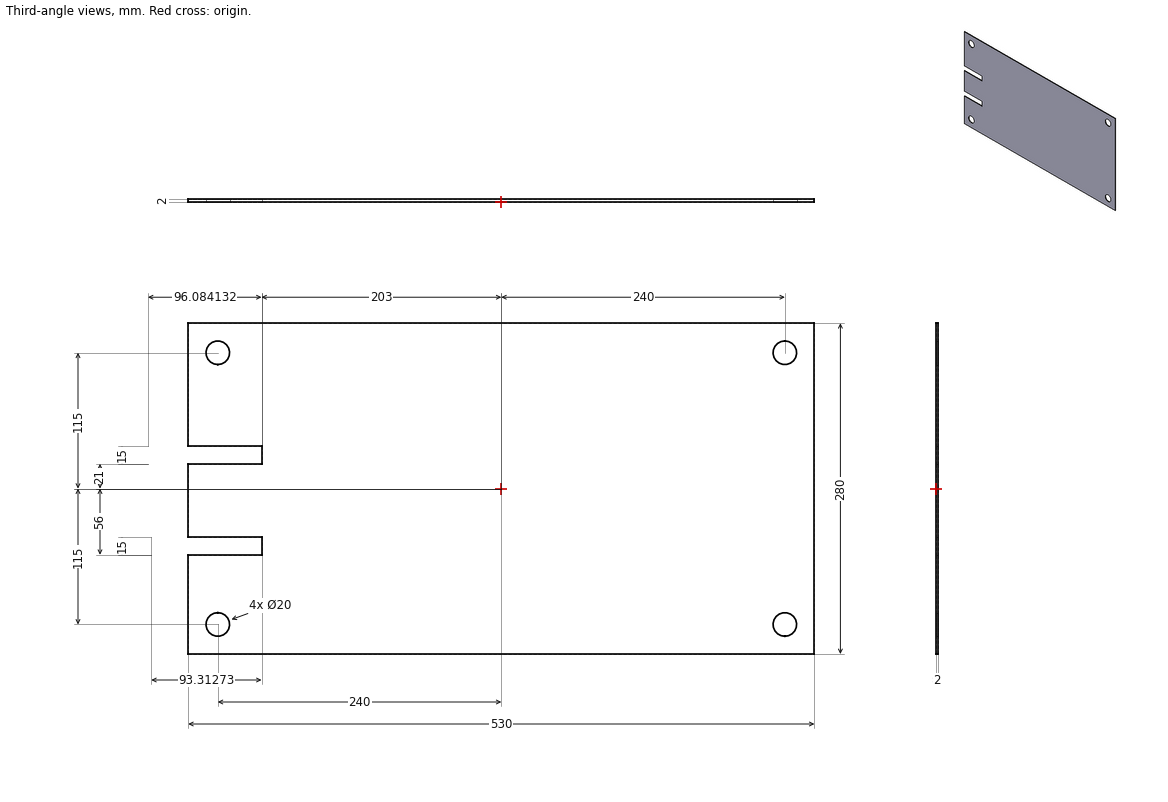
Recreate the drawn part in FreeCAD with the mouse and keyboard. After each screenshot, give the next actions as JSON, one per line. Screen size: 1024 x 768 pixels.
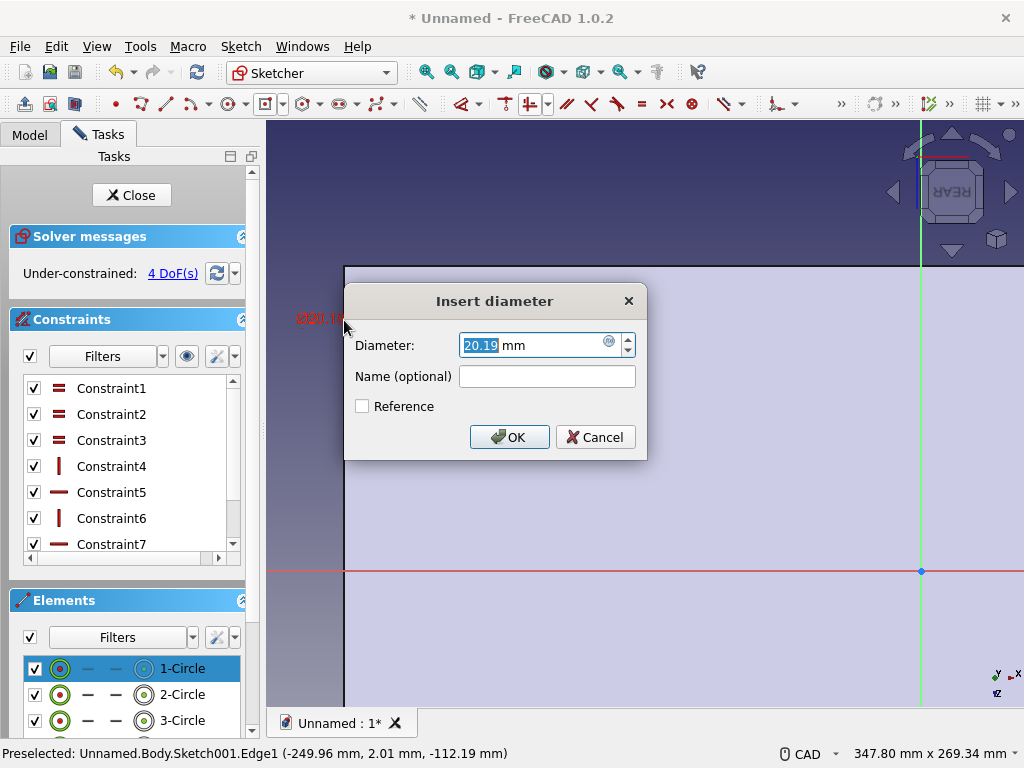
{"action": "type", "text": "20"}
{"action": "key", "text": "Return"}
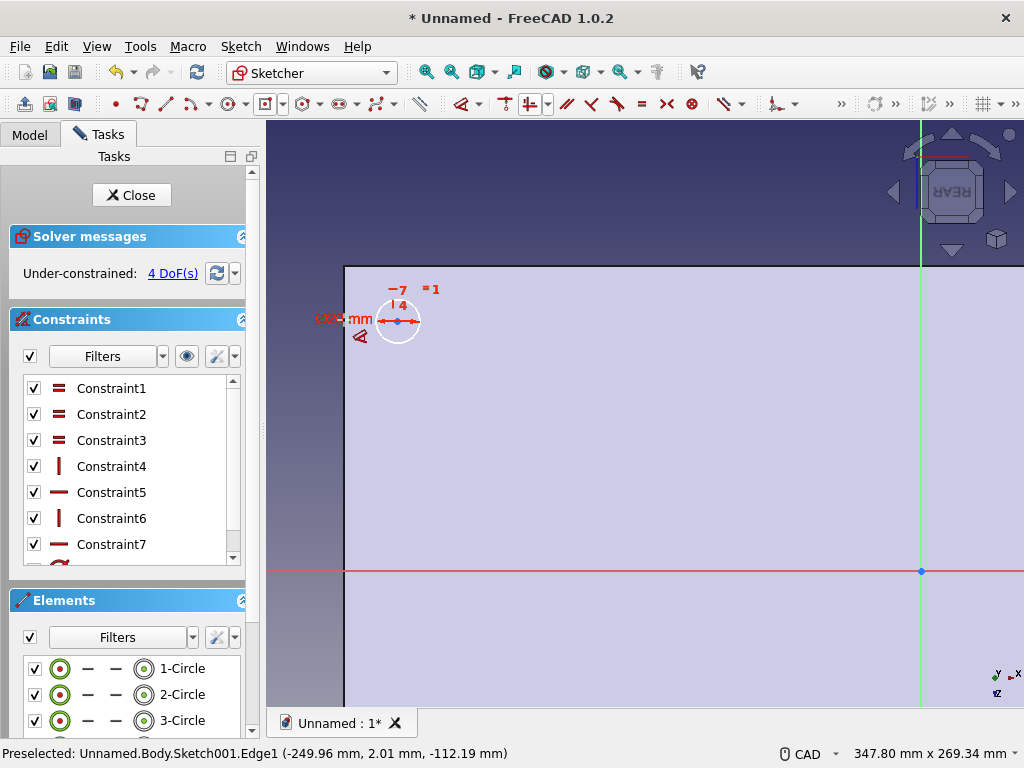
{"action": "left_click", "coordinate": [398, 321]}
{"action": "left_click", "coordinate": [628, 287]}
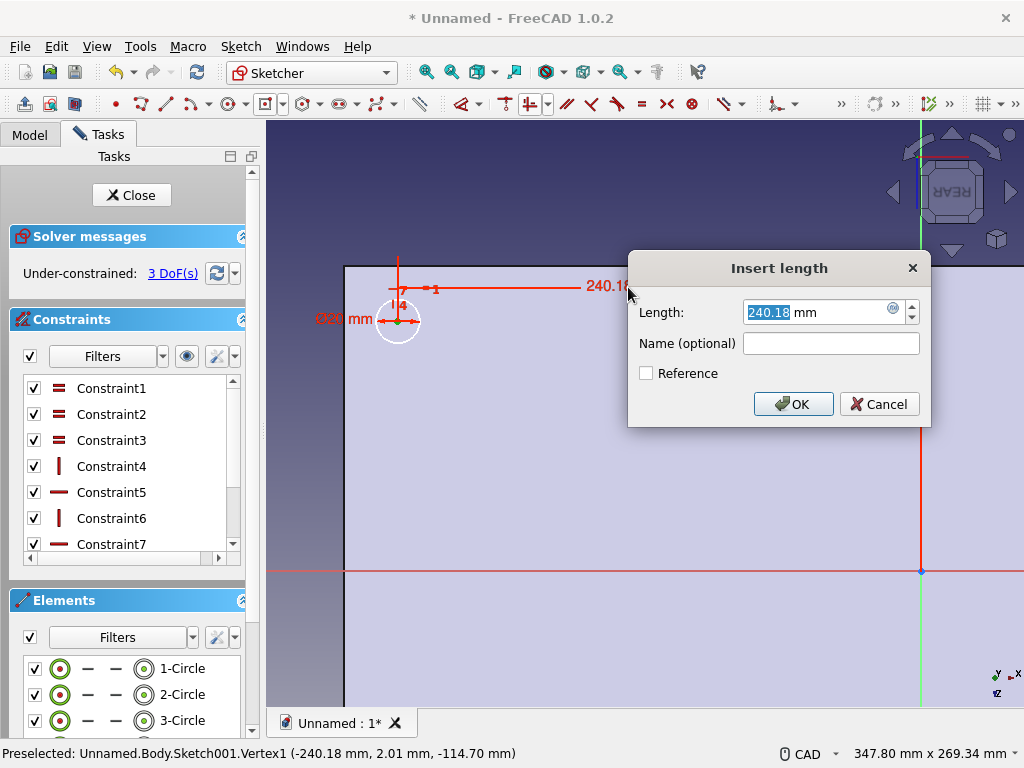
{"action": "type", "text": "240"}
{"action": "key", "text": "Return"}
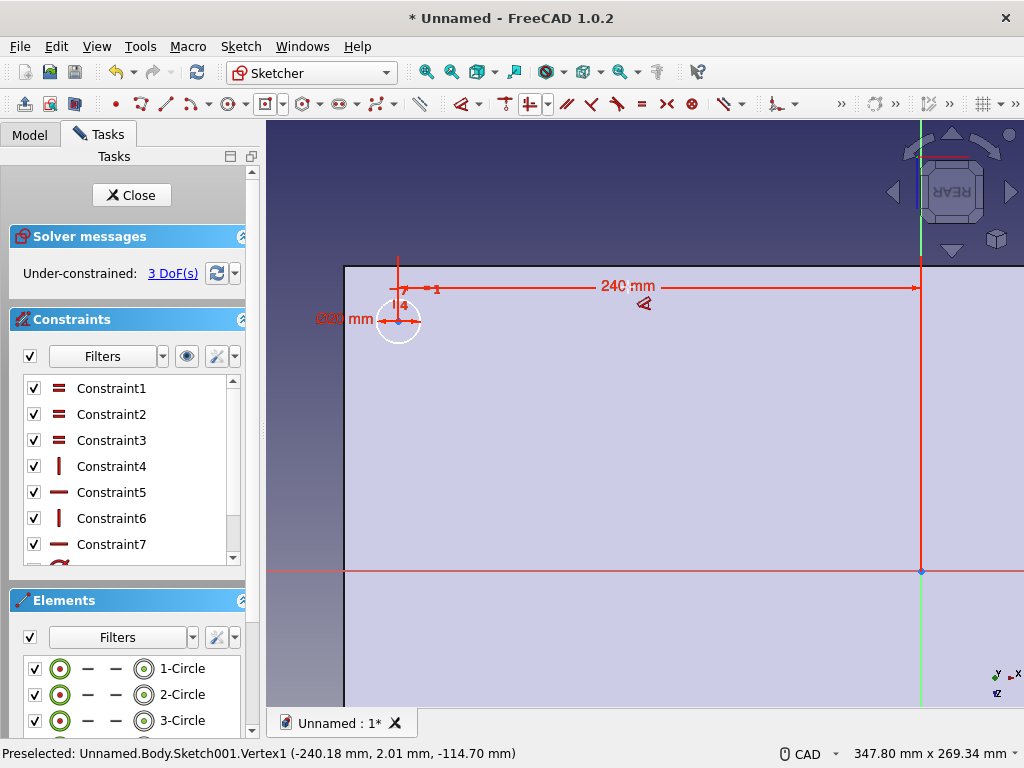
{"action": "left_click", "coordinate": [398, 321]}
{"action": "left_click", "coordinate": [364, 446]}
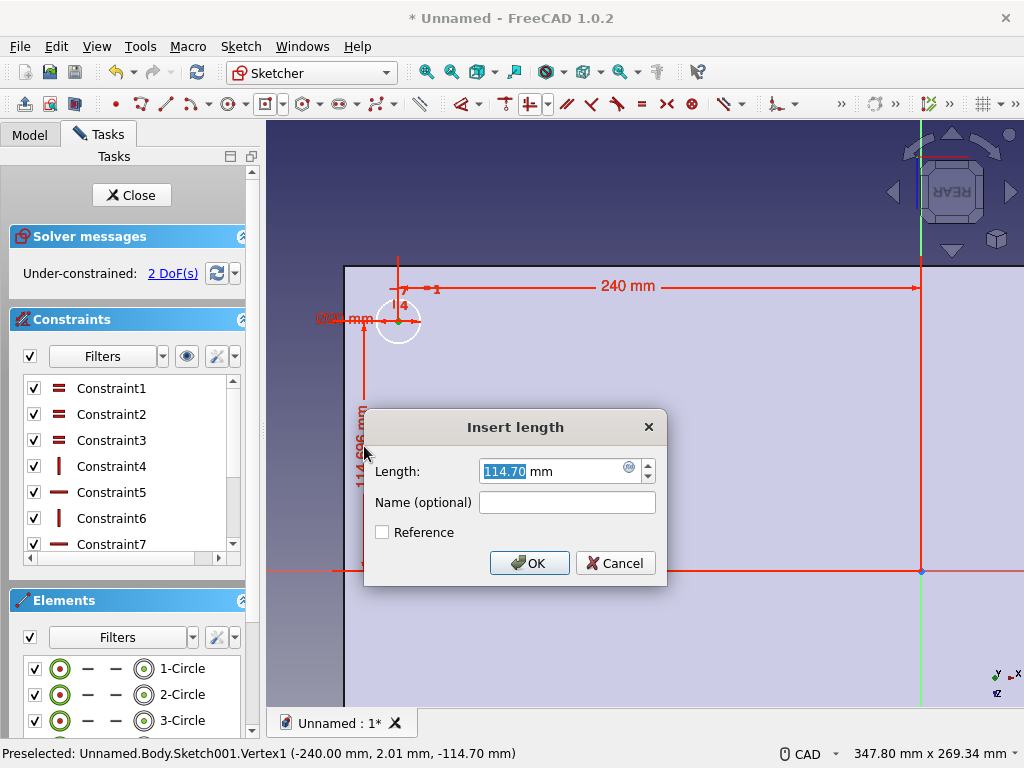
{"action": "type", "text": "115"}
{"action": "key", "text": "Return"}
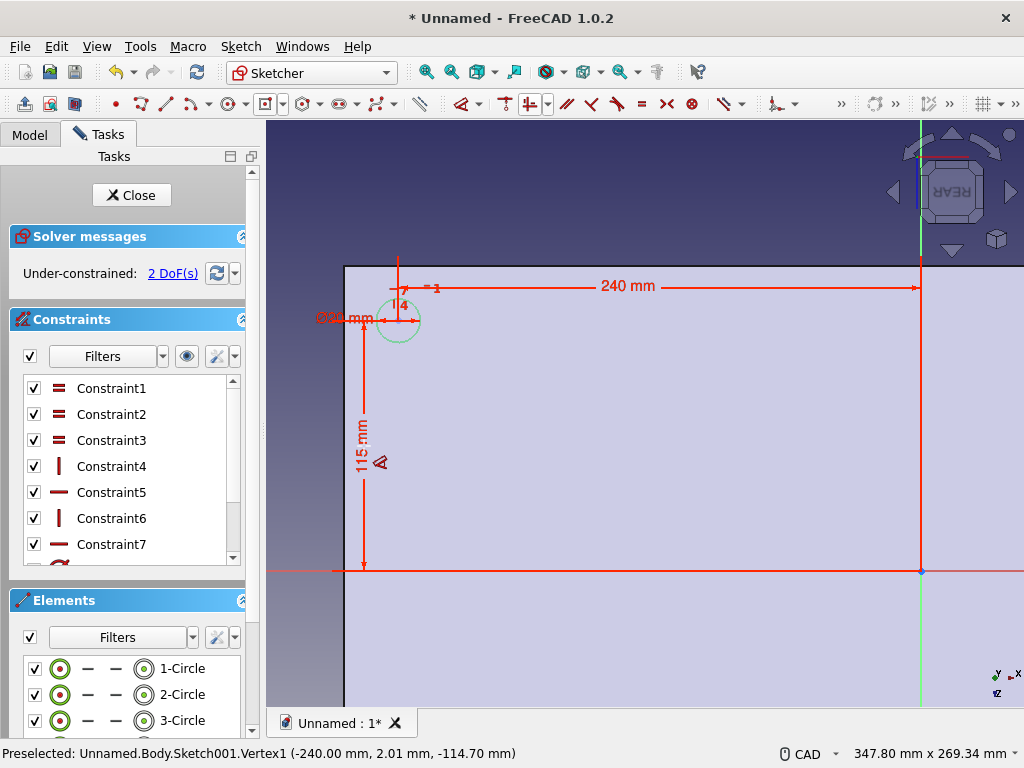
{"action": "scroll", "coordinate": [376, 322], "scroll_direction": "down", "scroll_amount": 5}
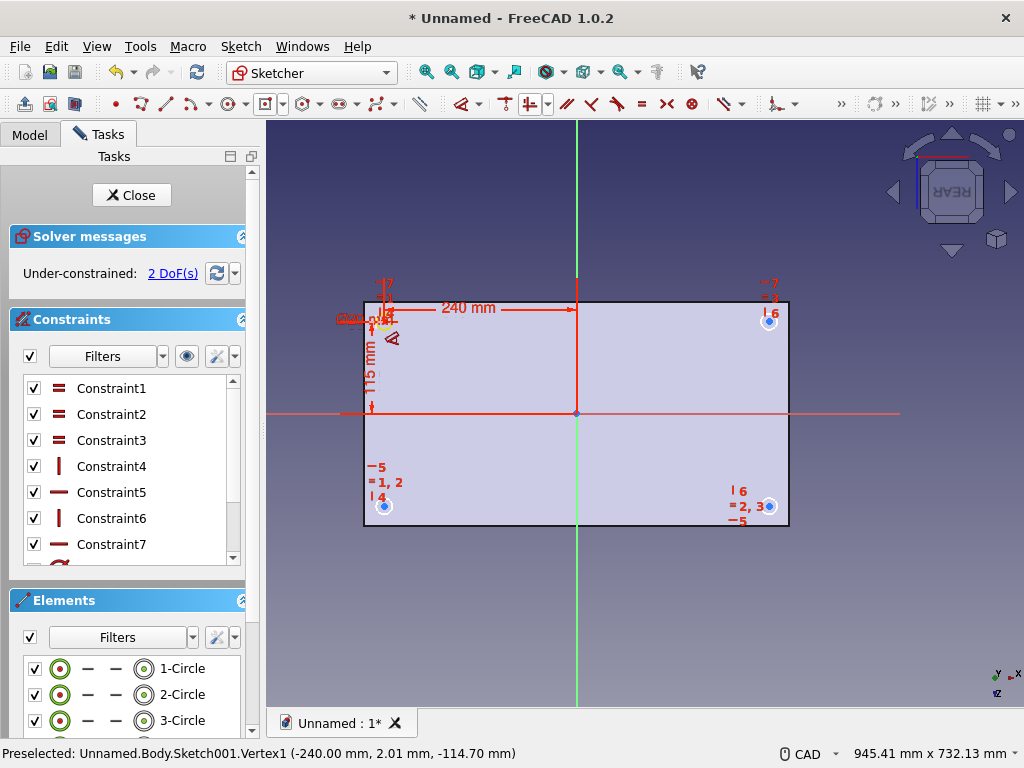
{"action": "left_click", "coordinate": [384, 506]}
{"action": "left_click", "coordinate": [350, 460]}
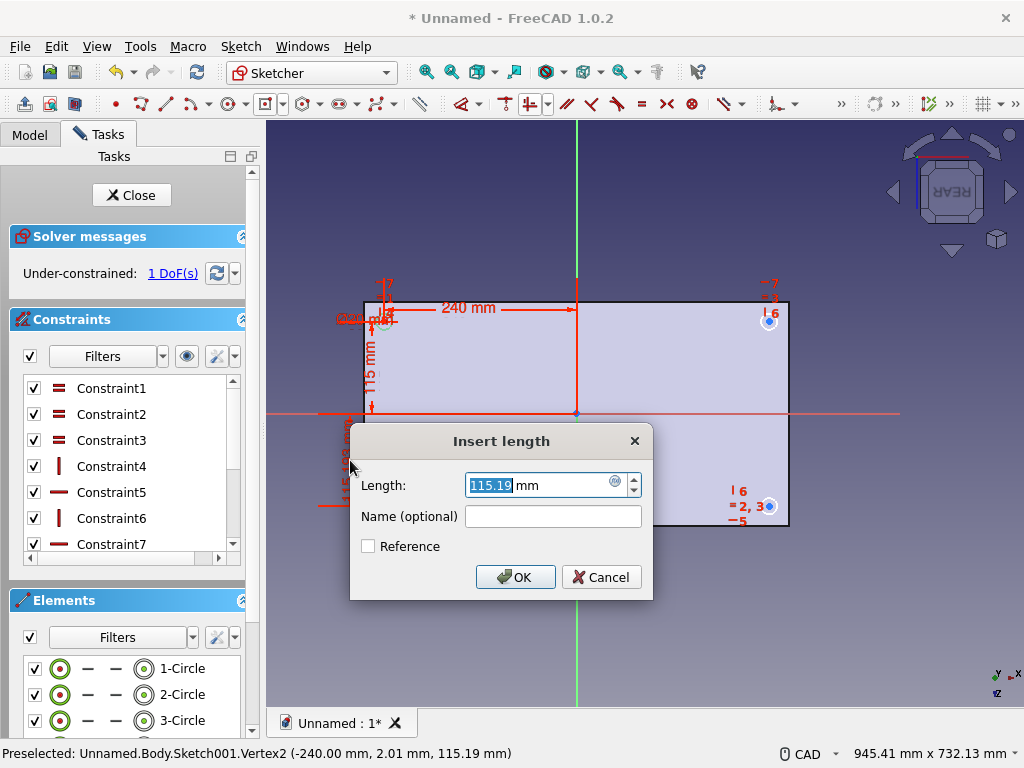
{"action": "type", "text": "115"}
{"action": "key", "text": "Return"}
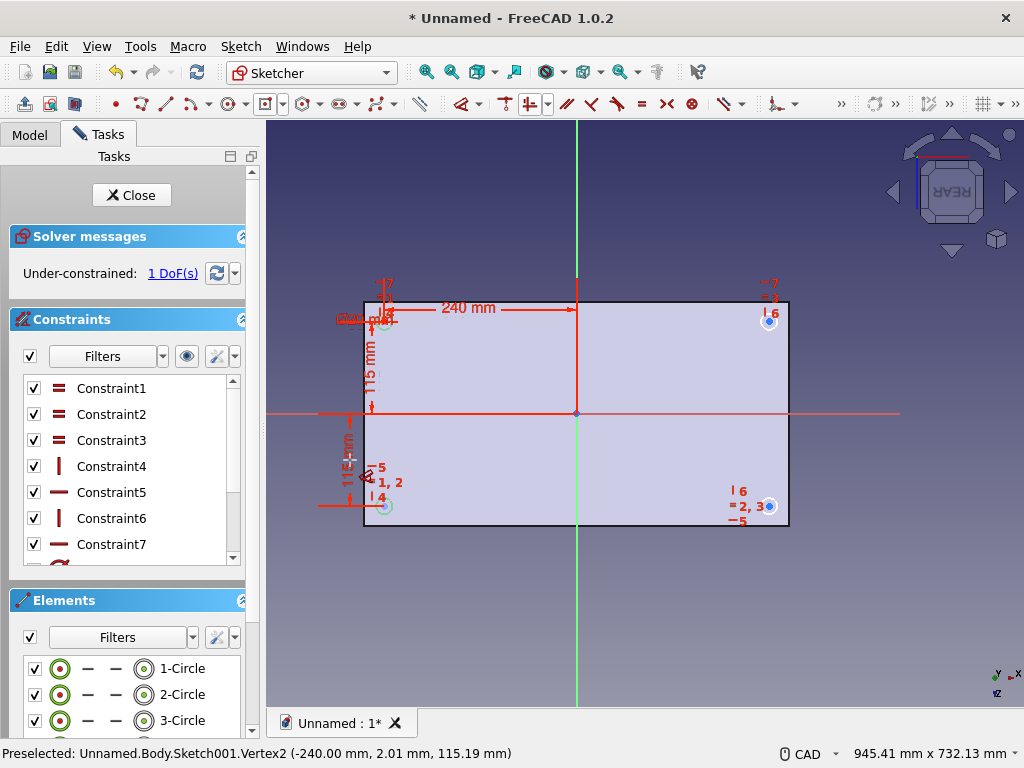
{"action": "left_click", "coordinate": [769, 506]}
{"action": "left_click", "coordinate": [673, 540]}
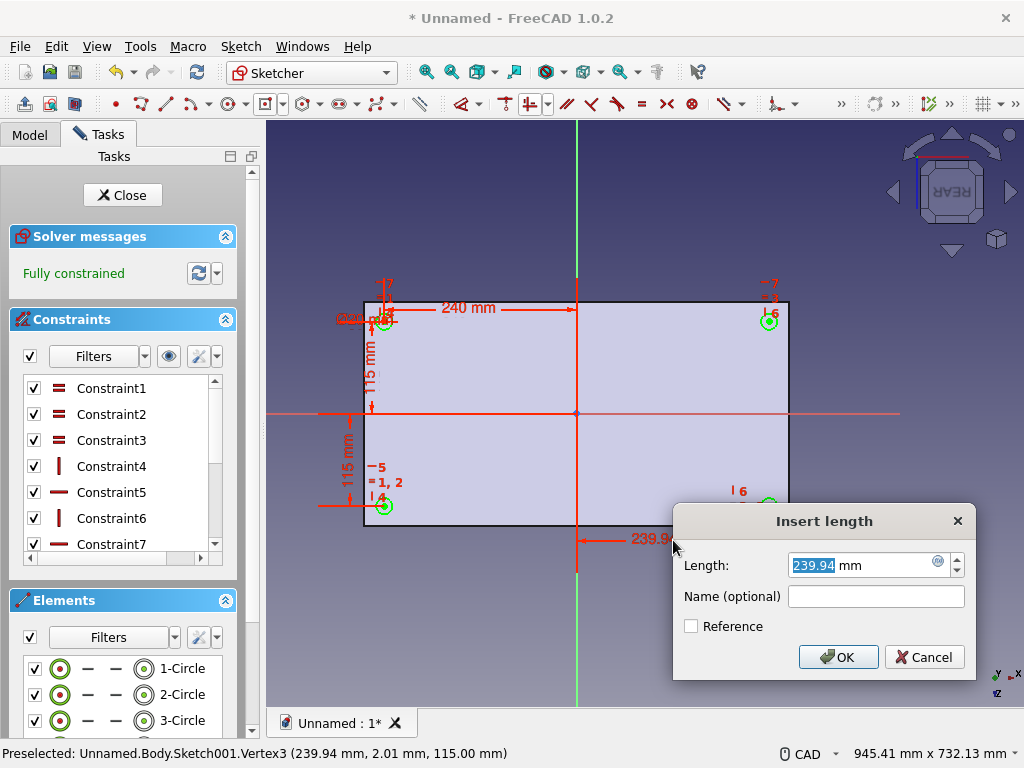
{"action": "type", "text": "240"}
{"action": "key", "text": "Return"}
{"action": "key", "text": "Escape"}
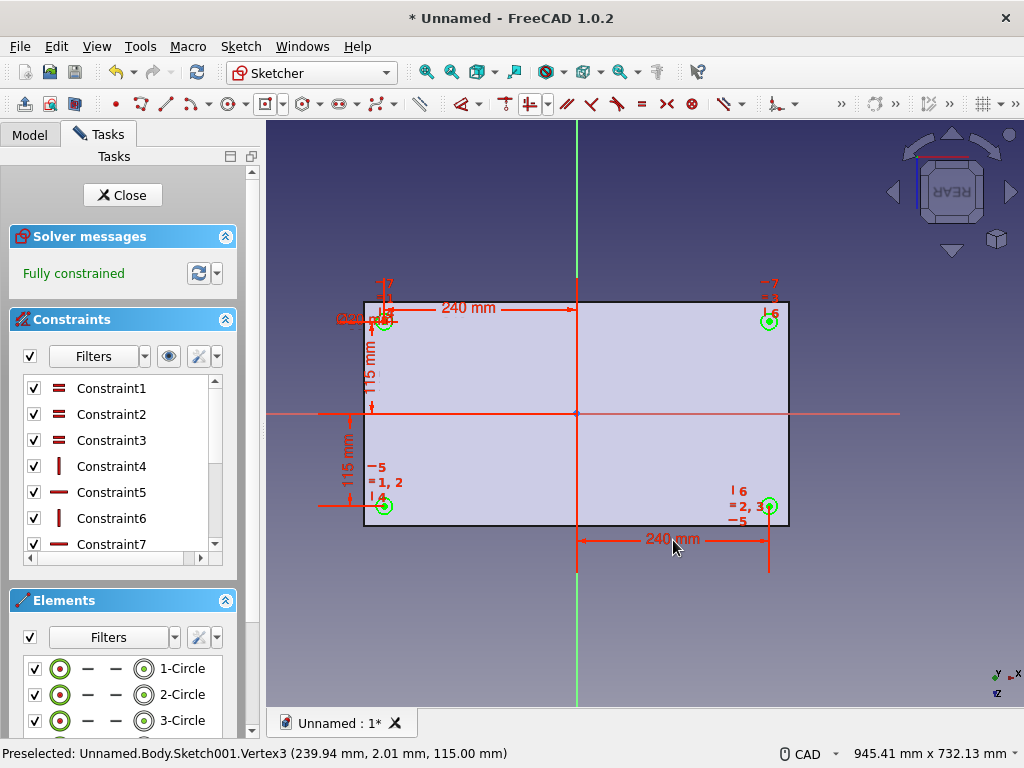
{"action": "left_click", "coordinate": [123, 195]}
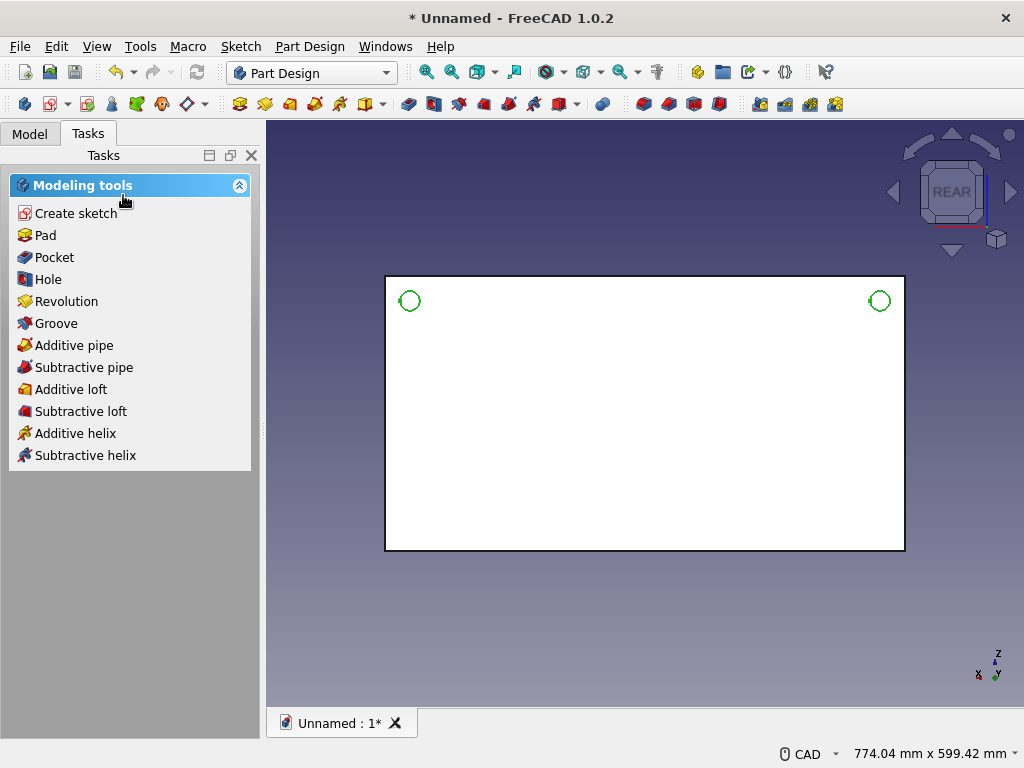
{"action": "left_click", "coordinate": [409, 104]}